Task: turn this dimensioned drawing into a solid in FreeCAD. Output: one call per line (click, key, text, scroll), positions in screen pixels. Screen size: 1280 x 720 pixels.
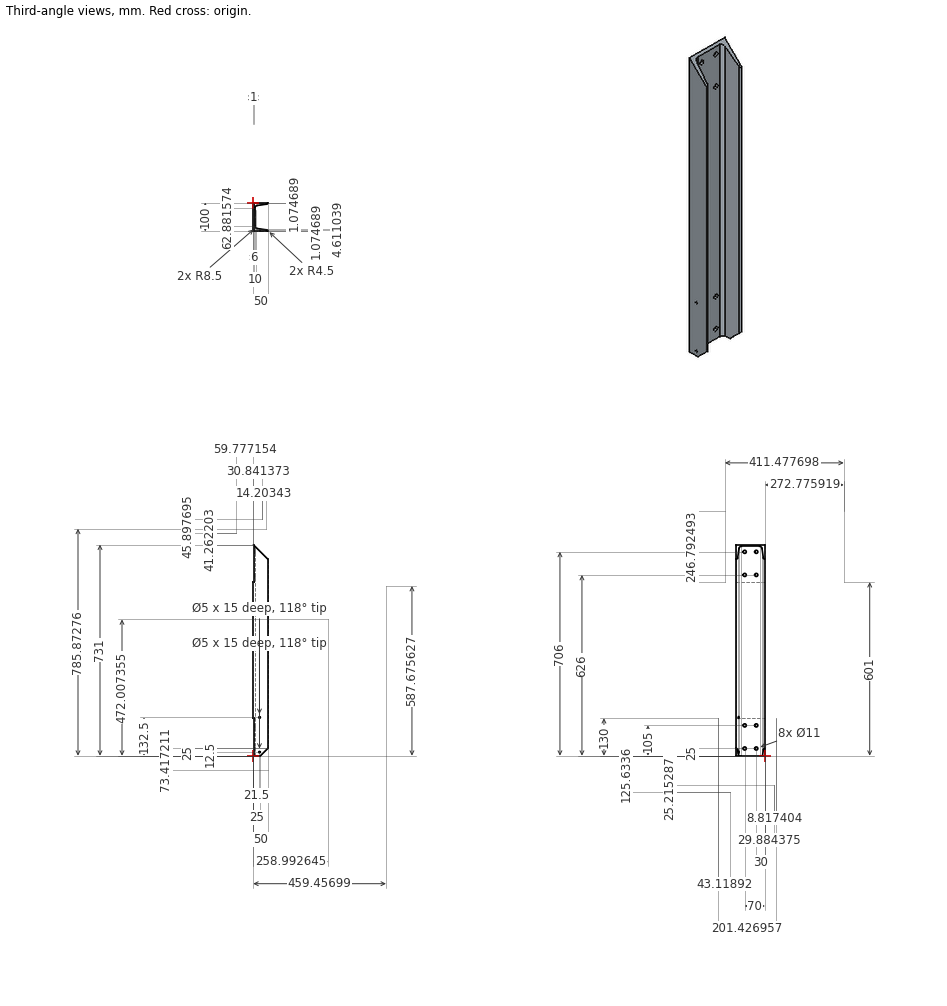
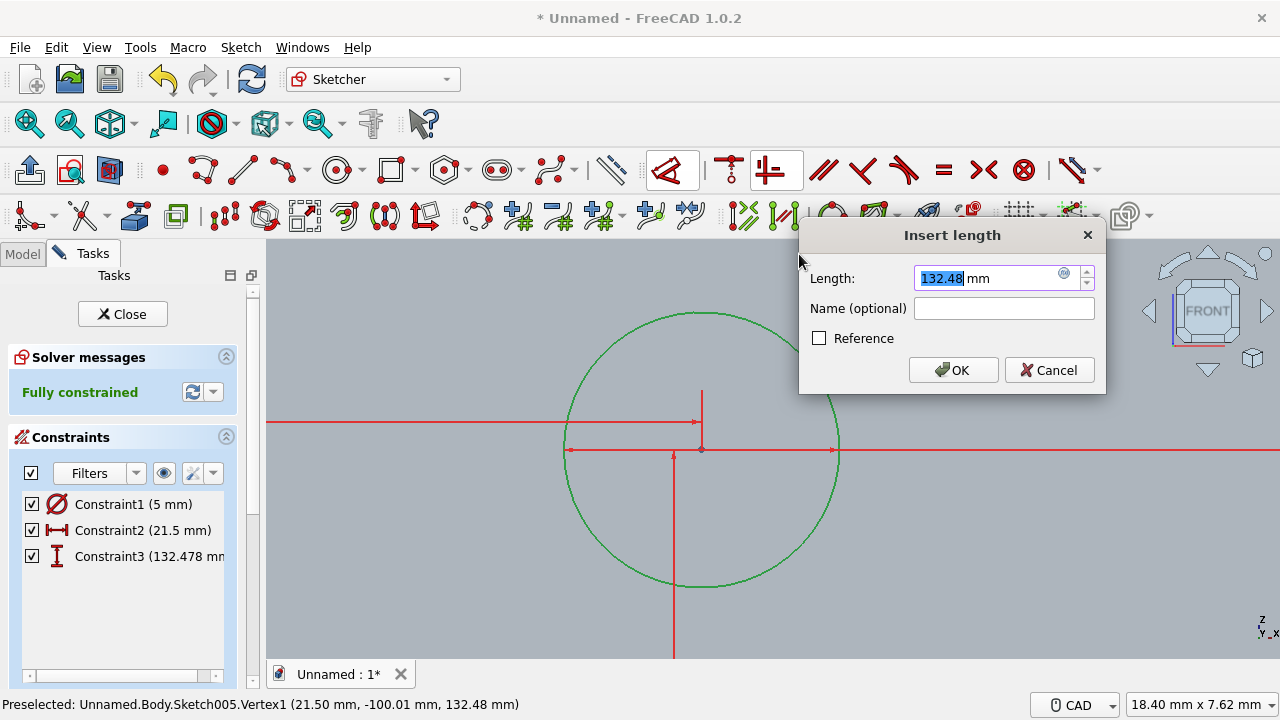
text(132.5)
key(Return)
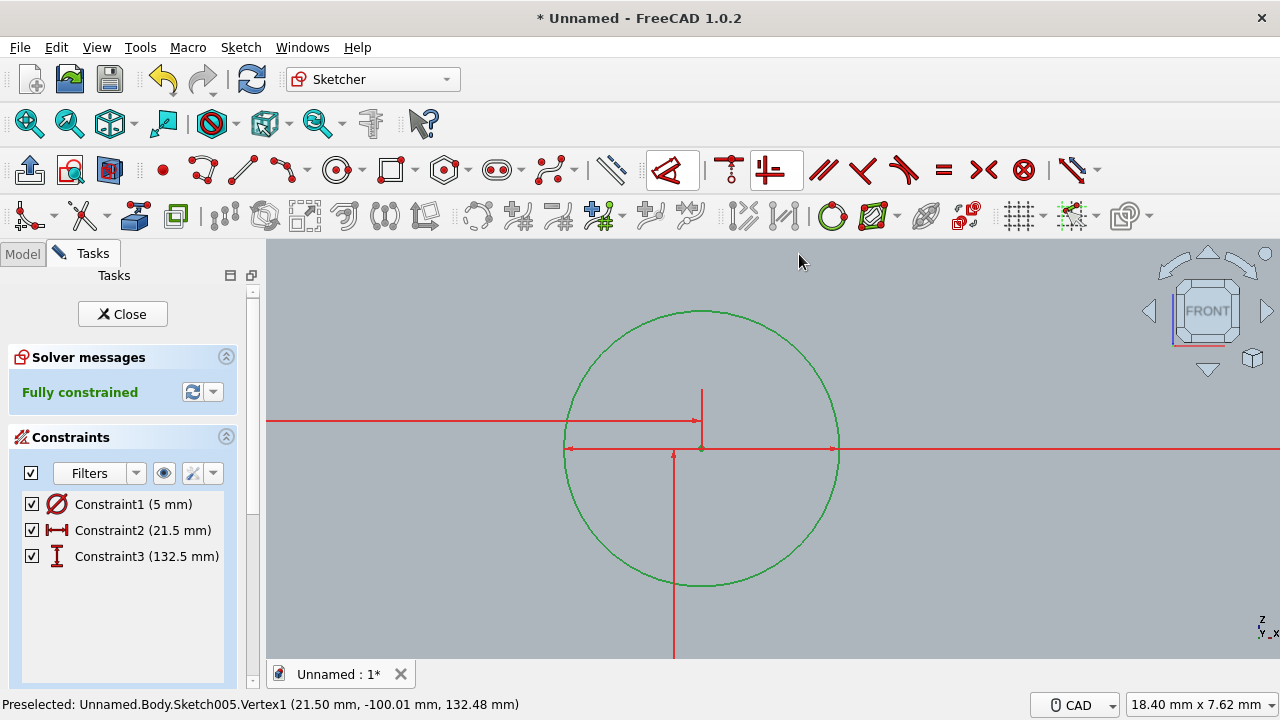
click(123, 314)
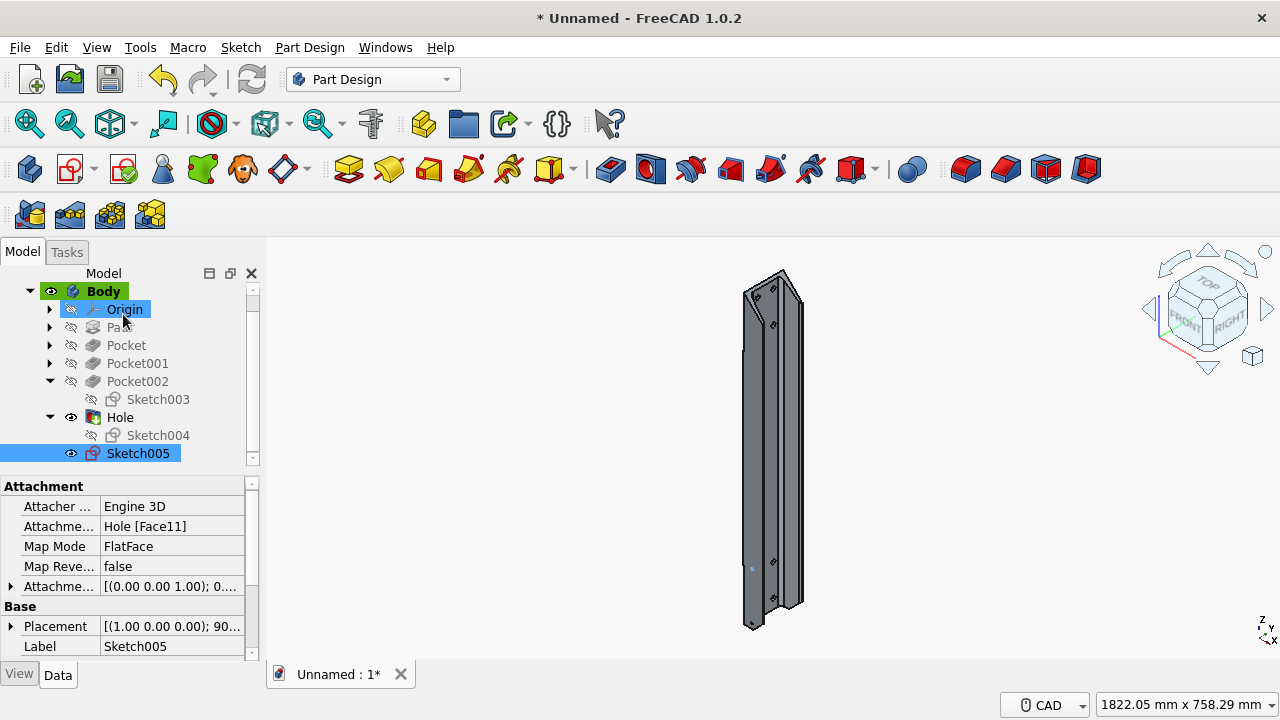
click(652, 170)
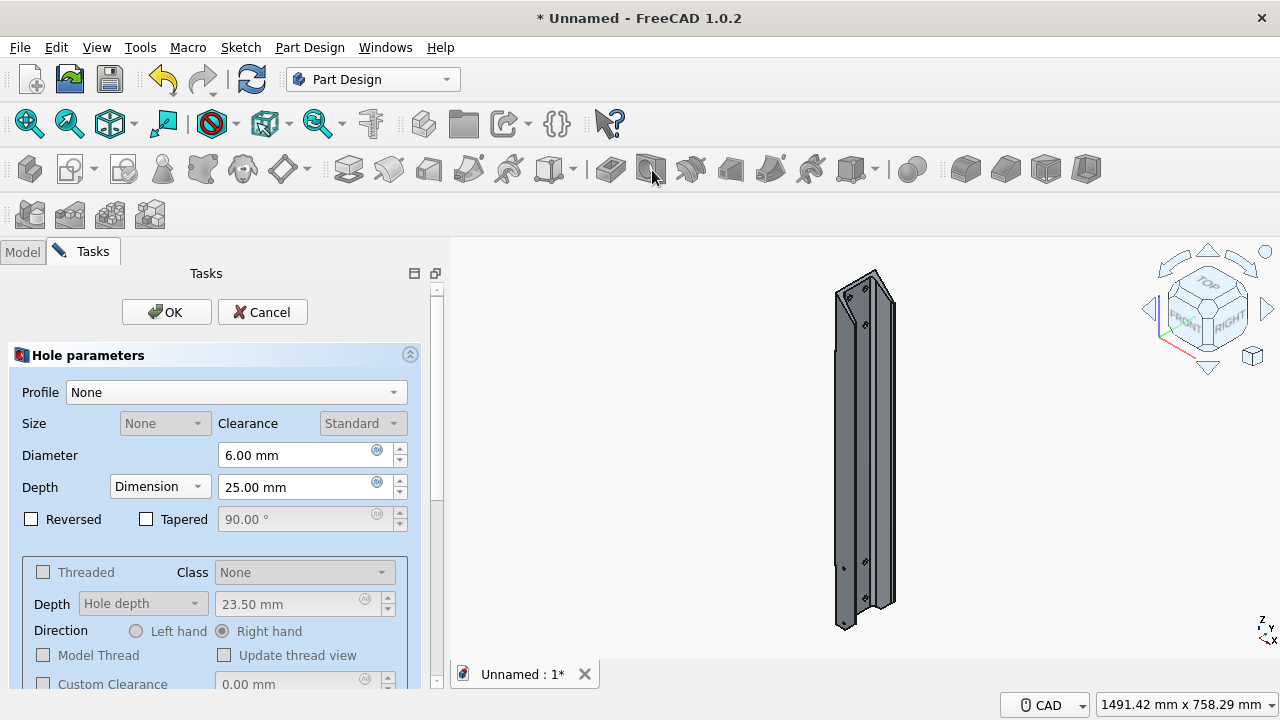
triple_click(305, 455)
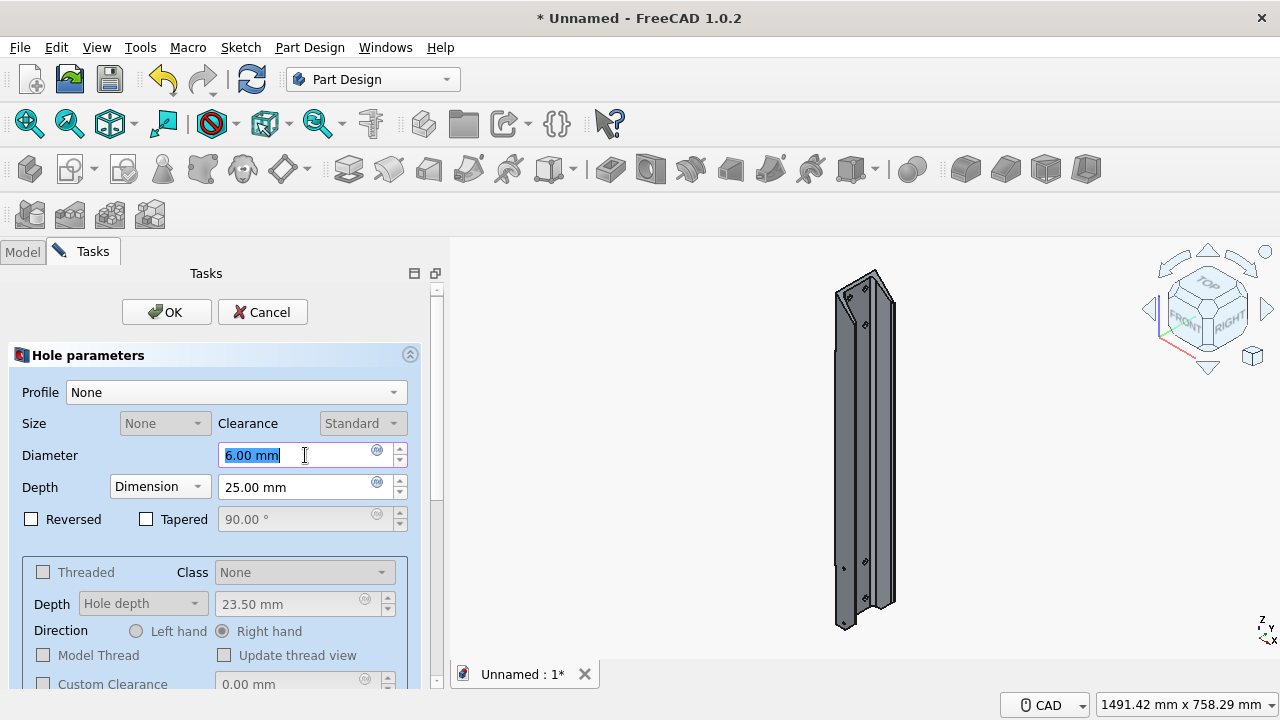
text(5)
key(Tab)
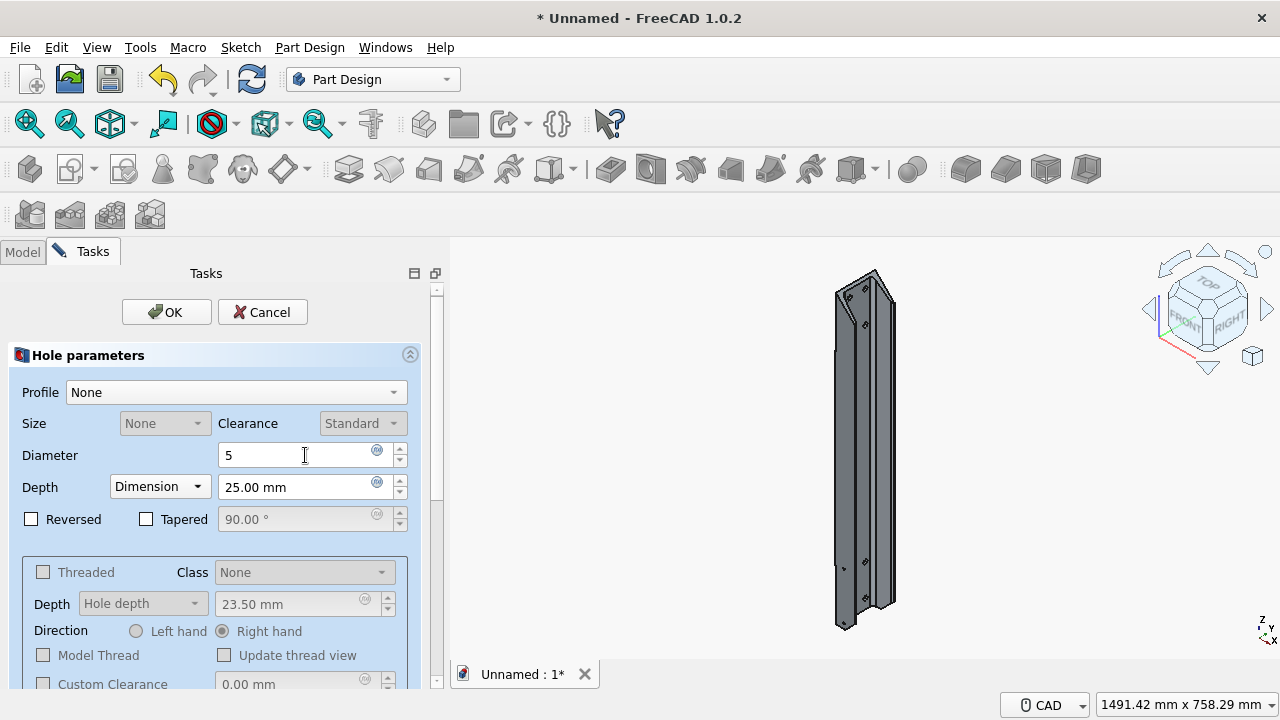
triple_click(305, 487)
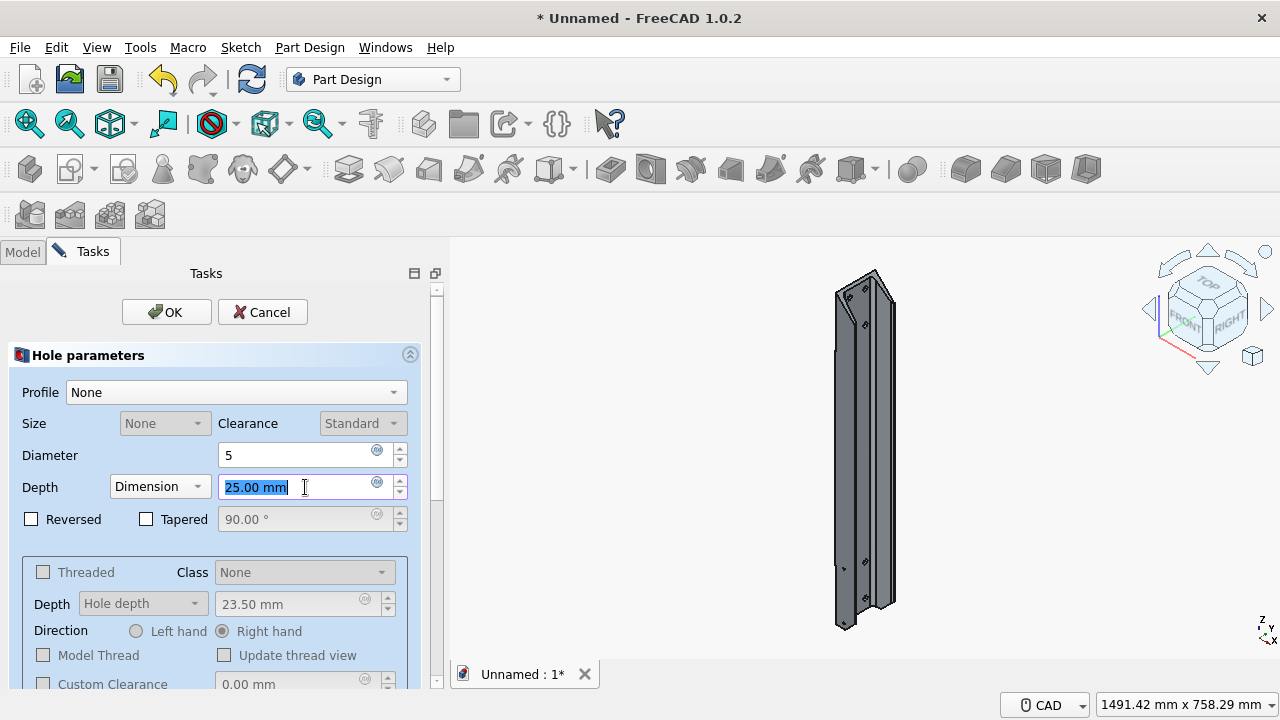
text(15)
key(Tab)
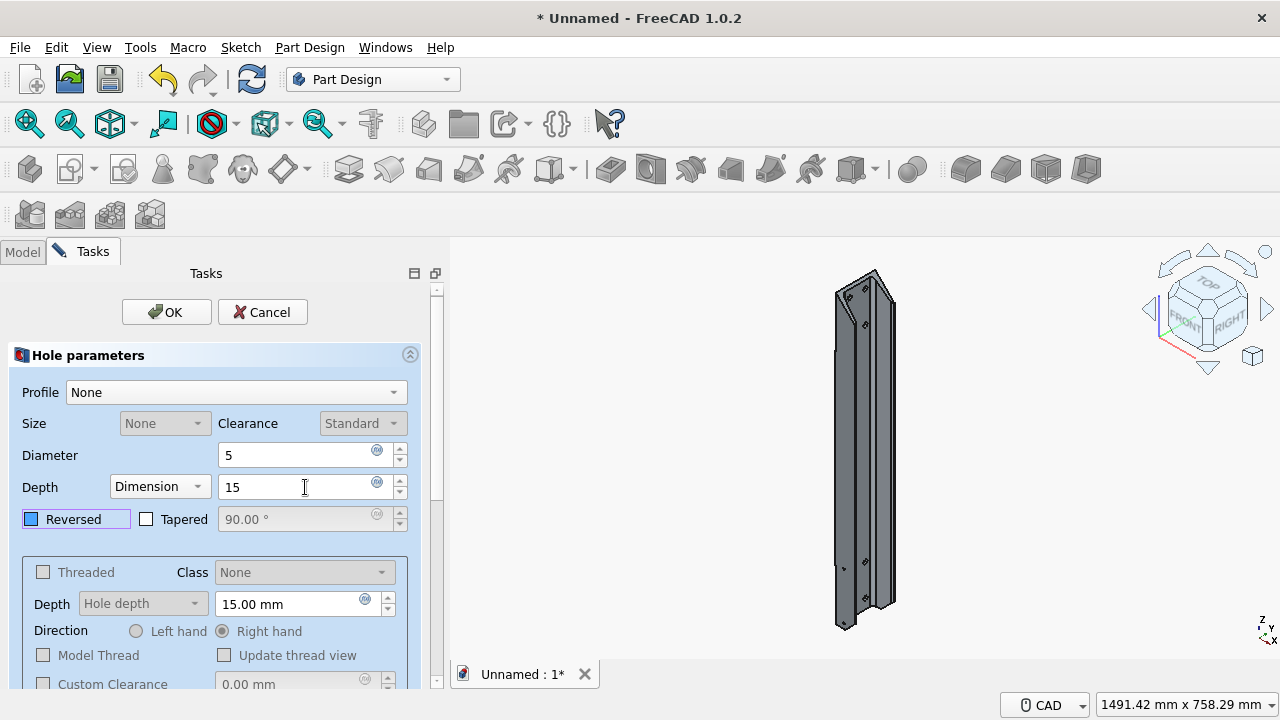
click(167, 312)